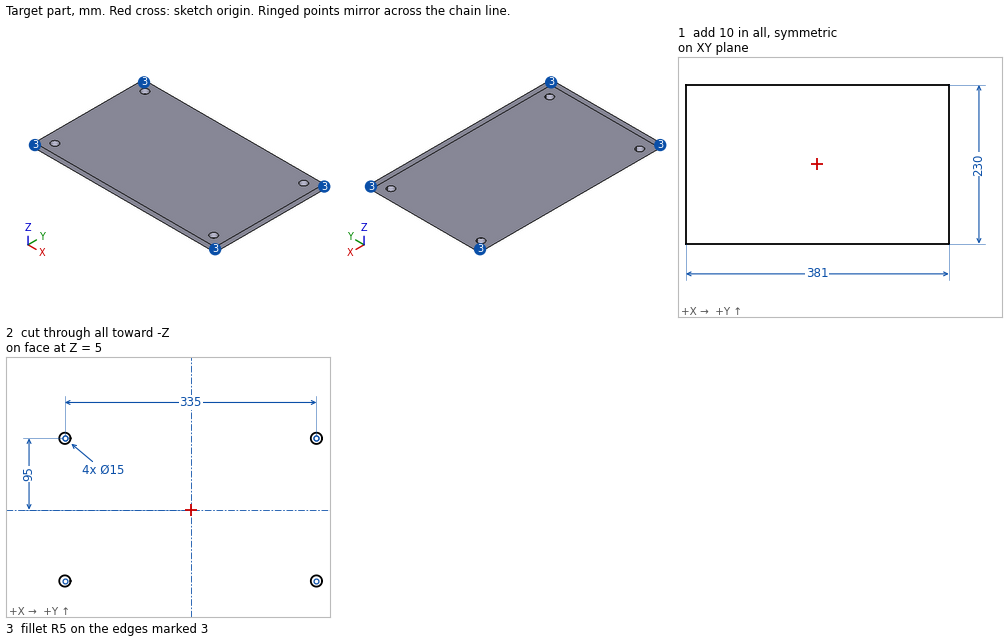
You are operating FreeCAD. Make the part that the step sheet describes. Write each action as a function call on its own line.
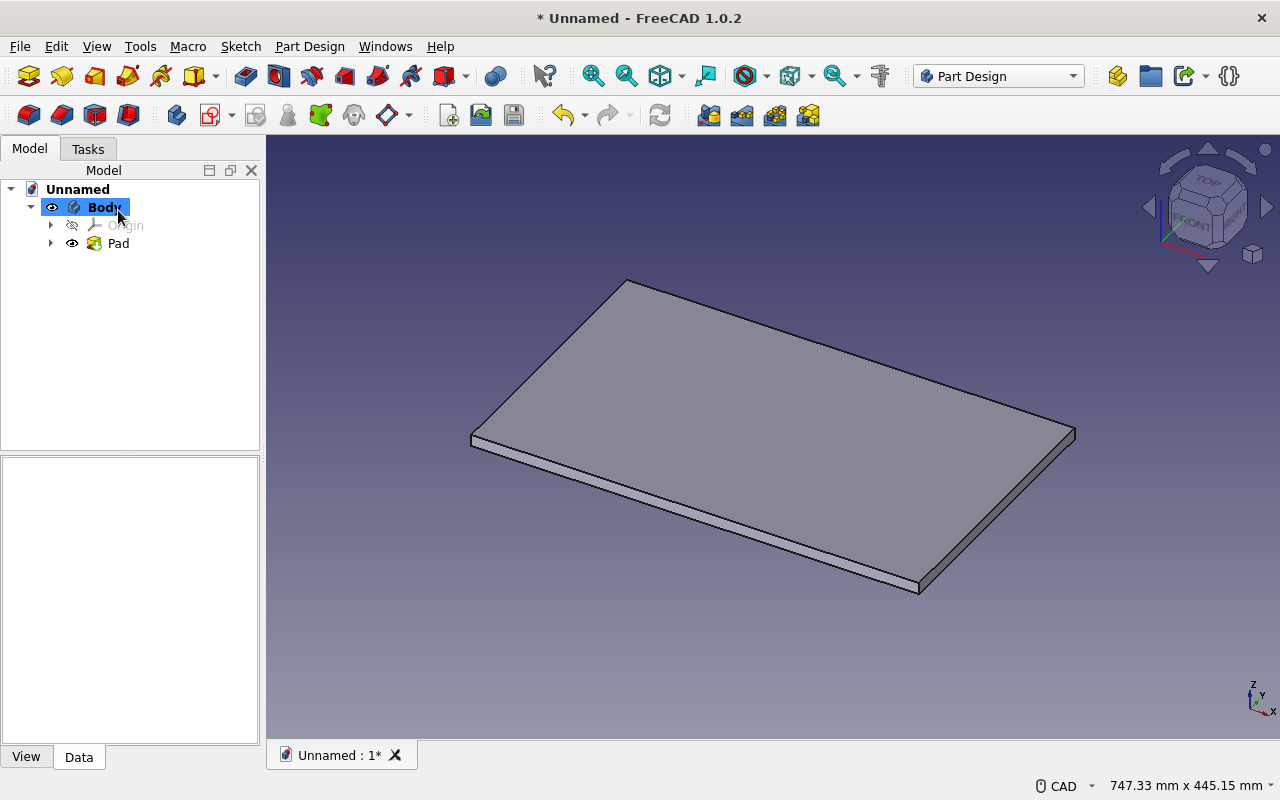
click(837, 452)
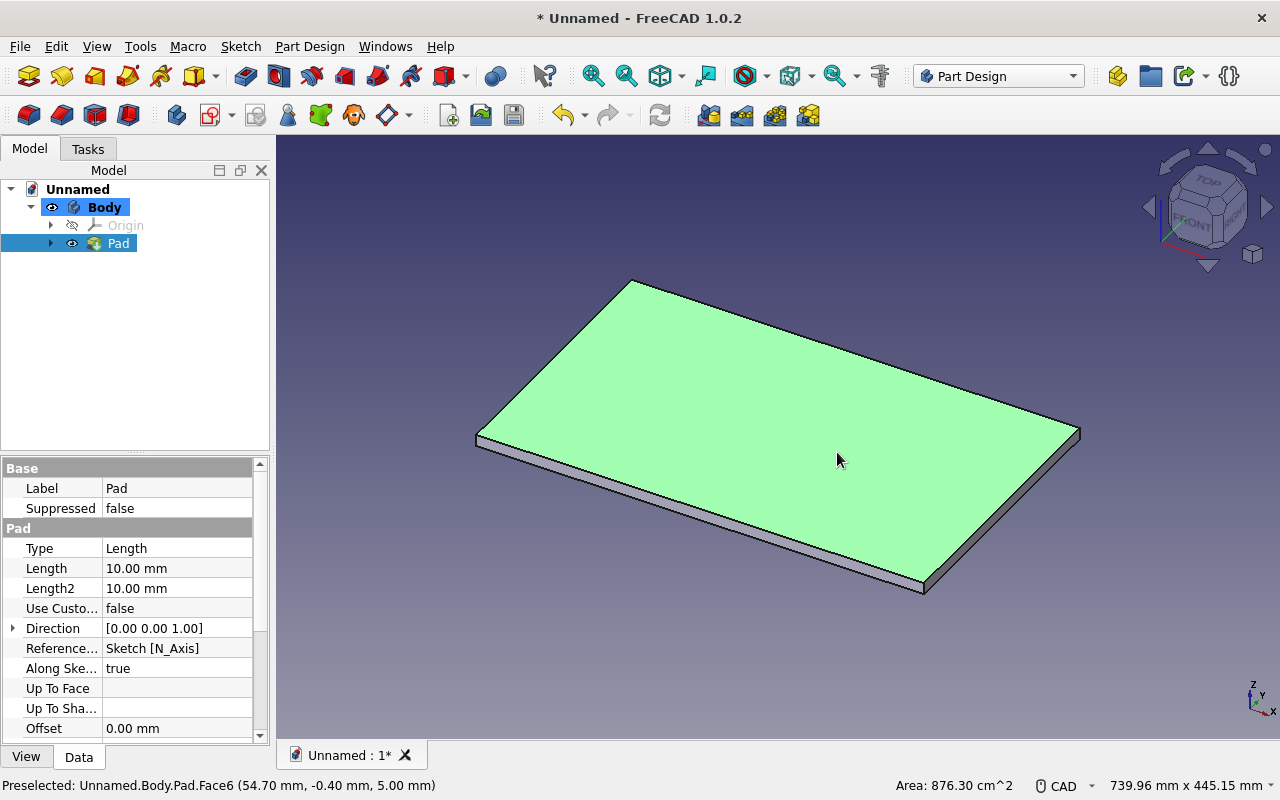
click(210, 116)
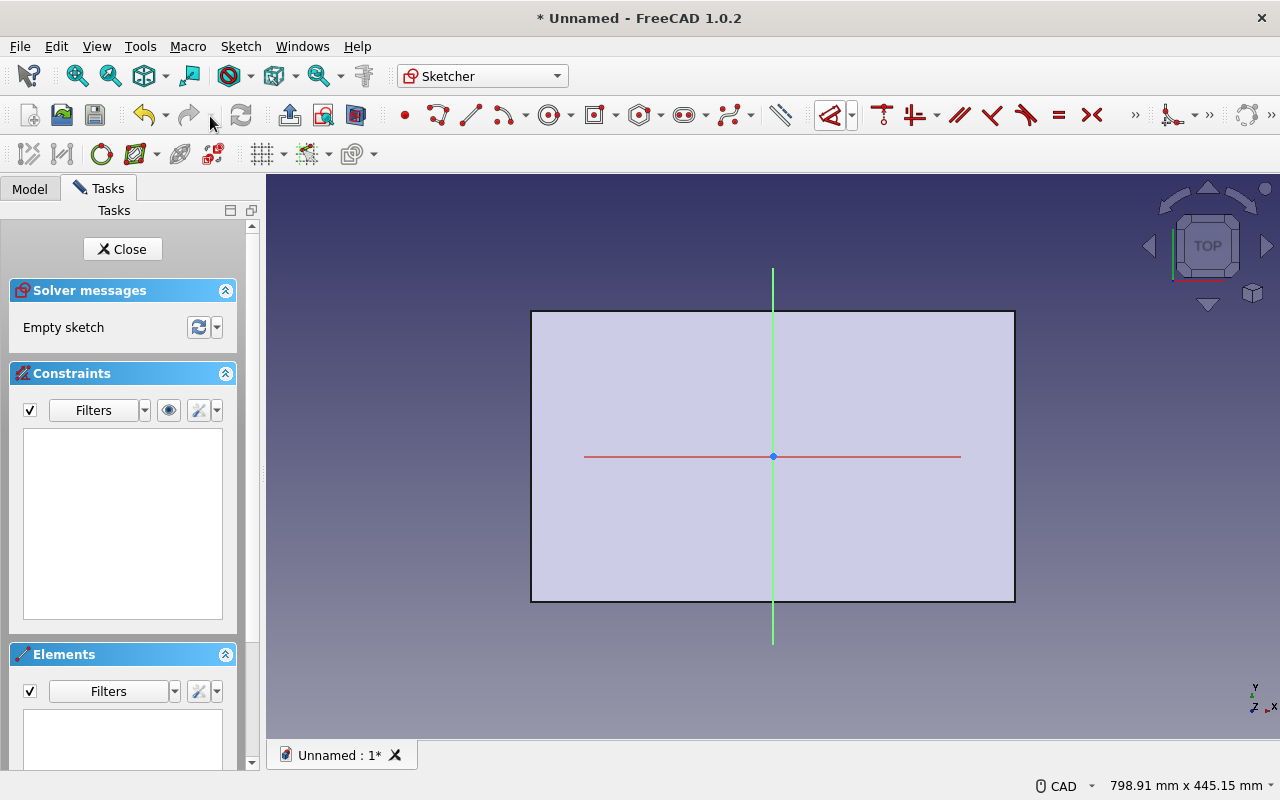
click(548, 116)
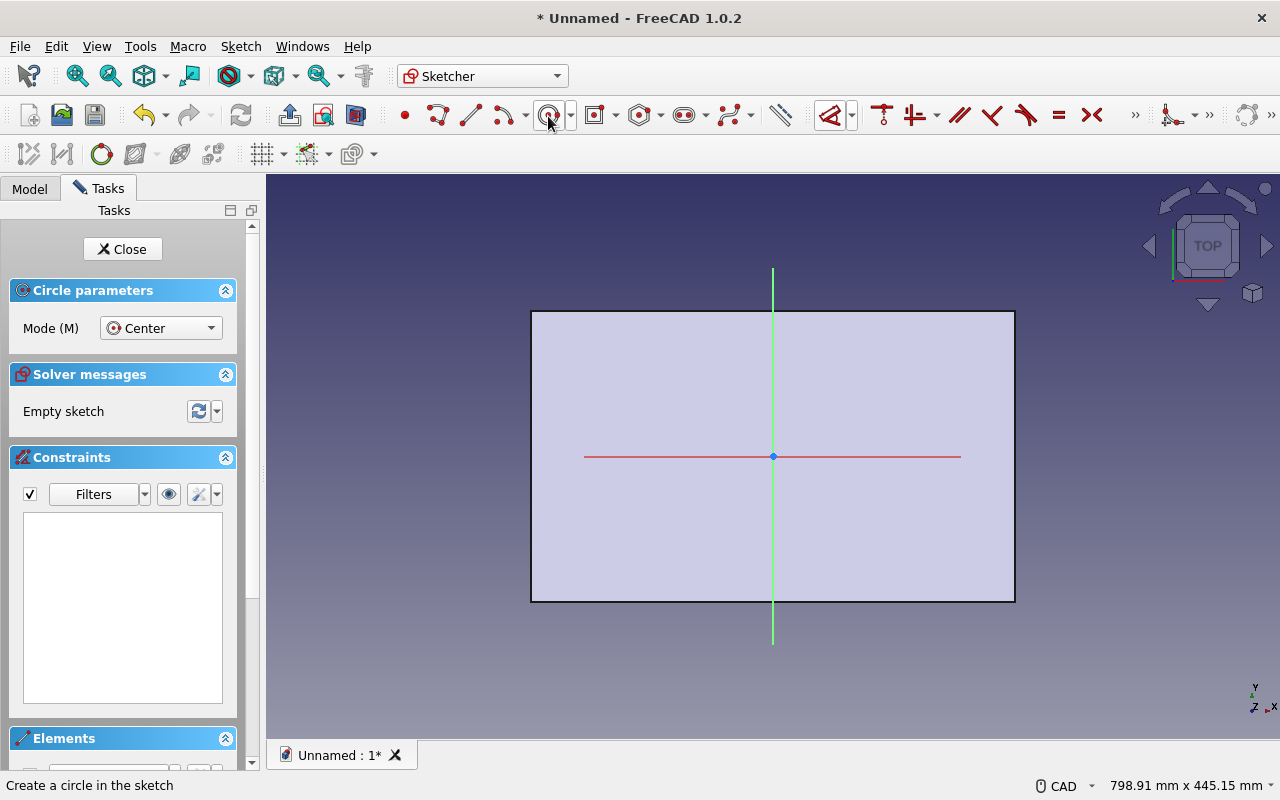
scroll(560, 336, up, 5)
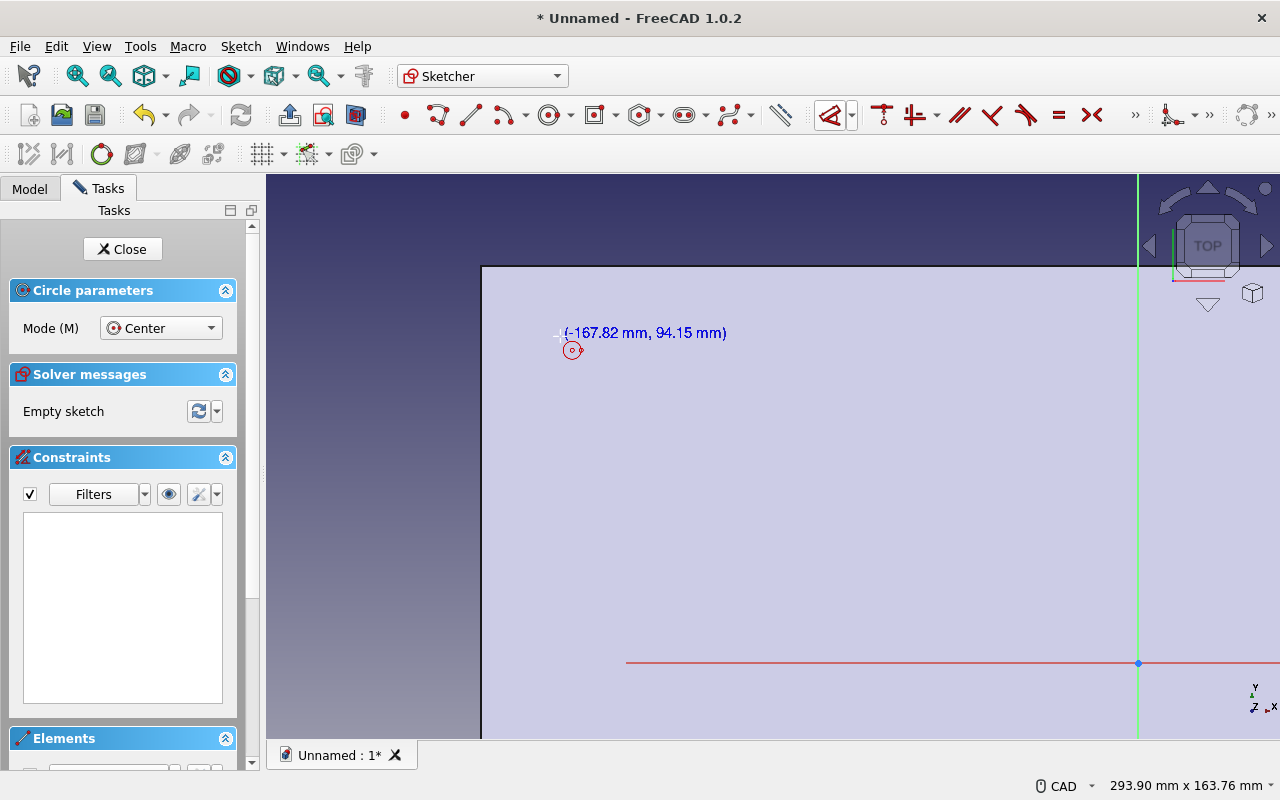
click(561, 335)
click(579, 317)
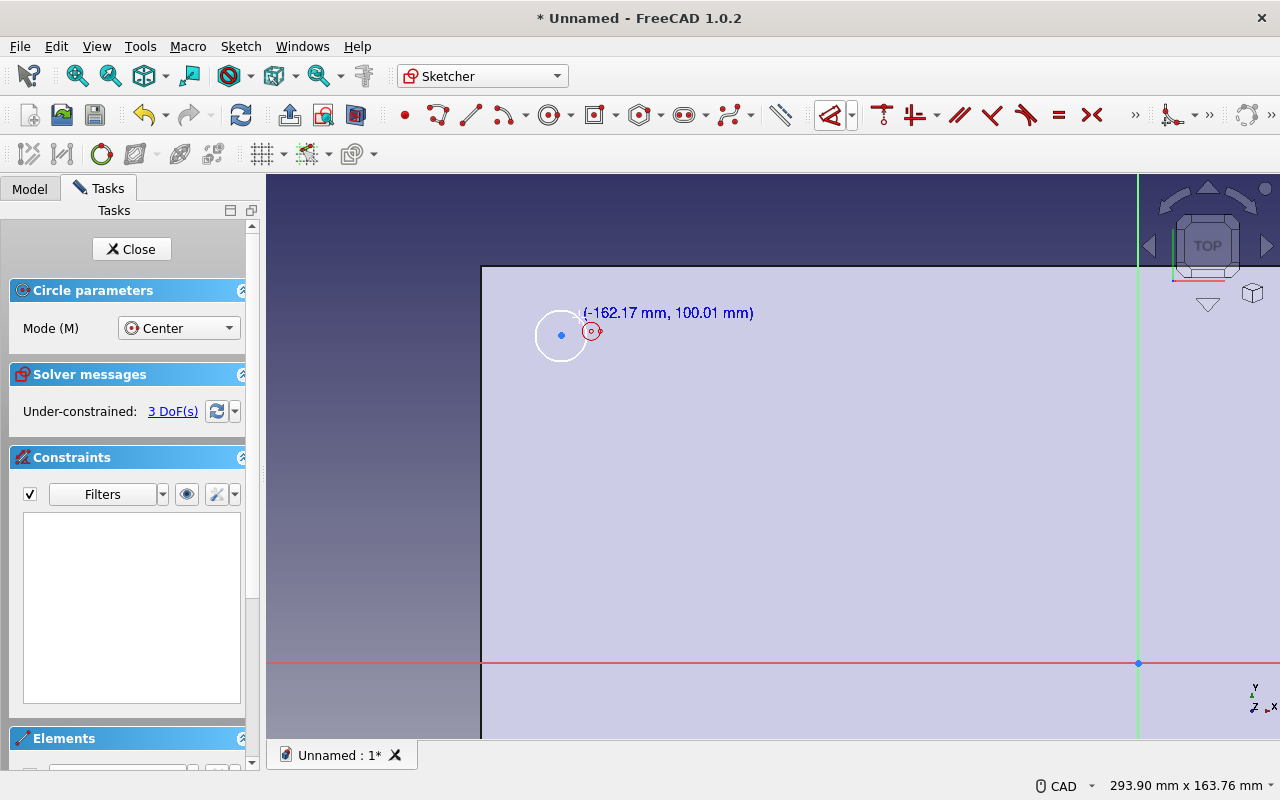
scroll(350, 288, down, 4)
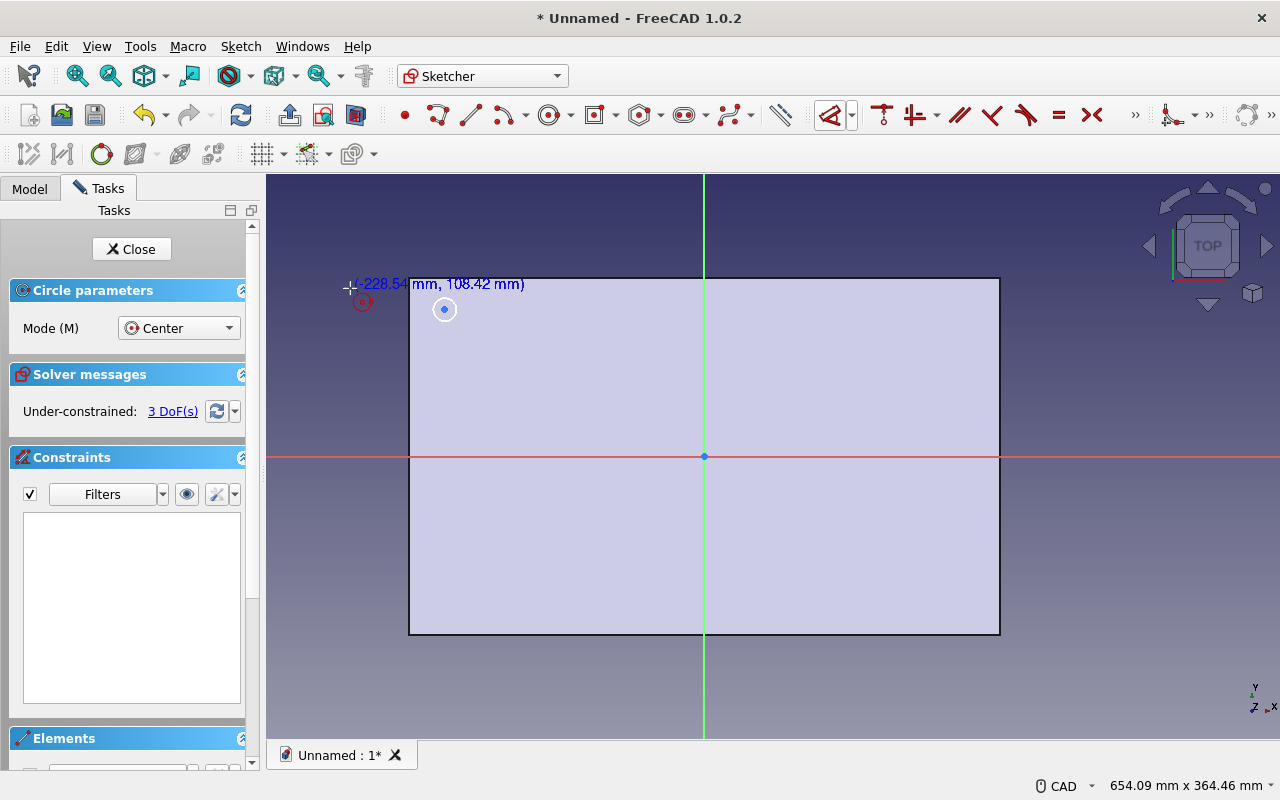
scroll(964, 309, up, 4)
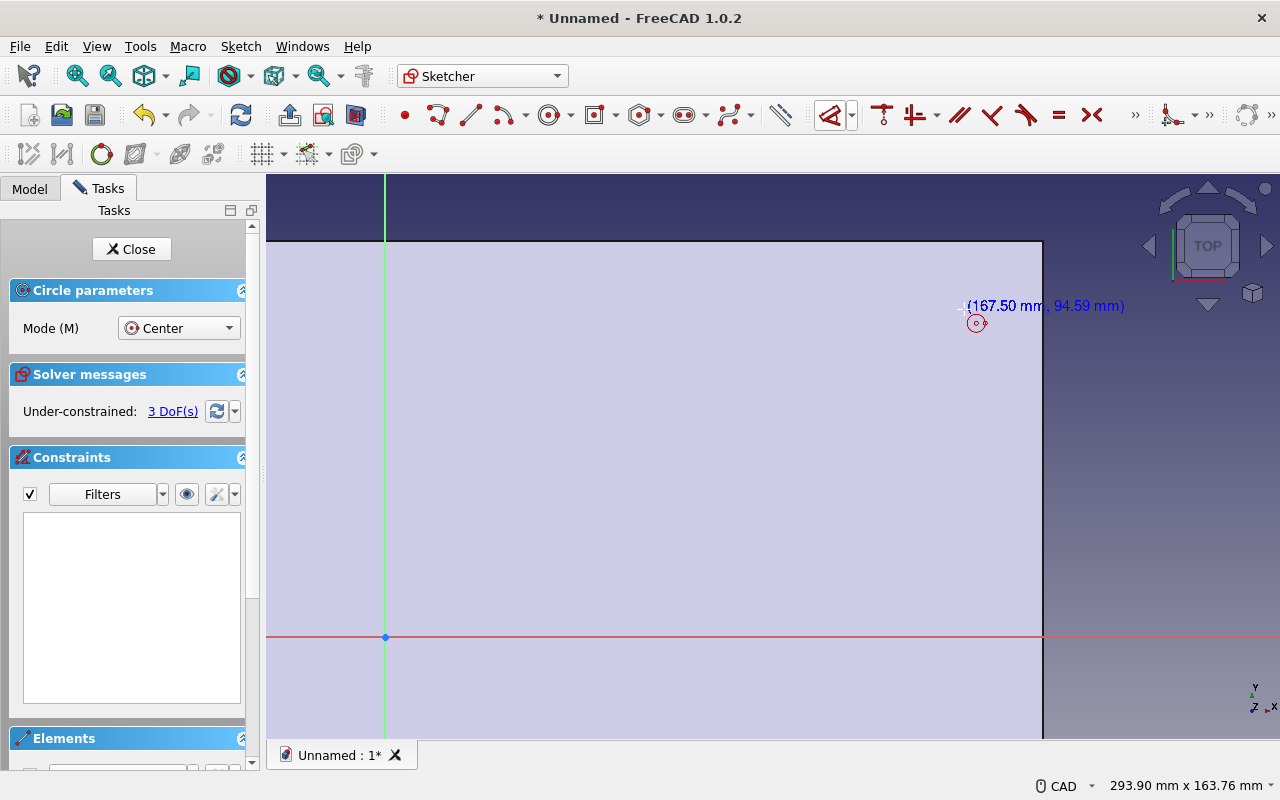
click(963, 310)
click(981, 291)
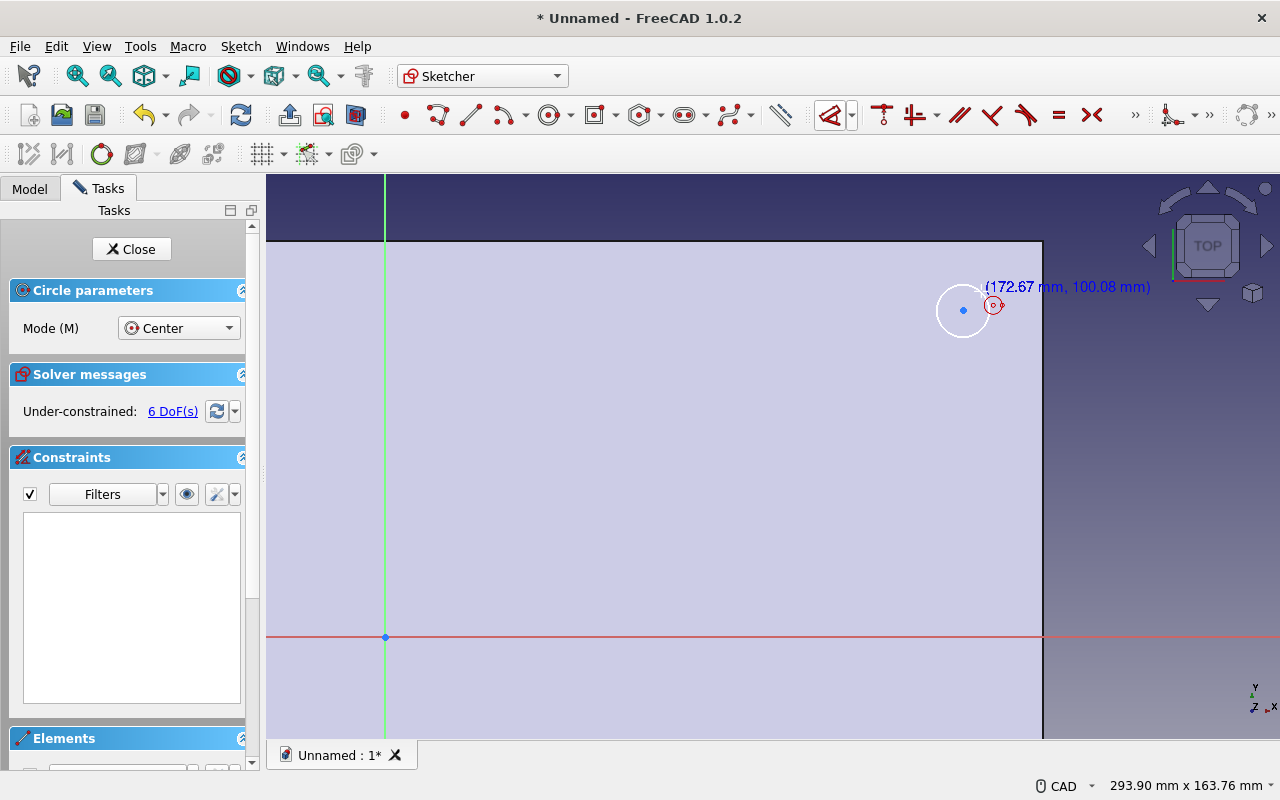
scroll(965, 309, down, 4)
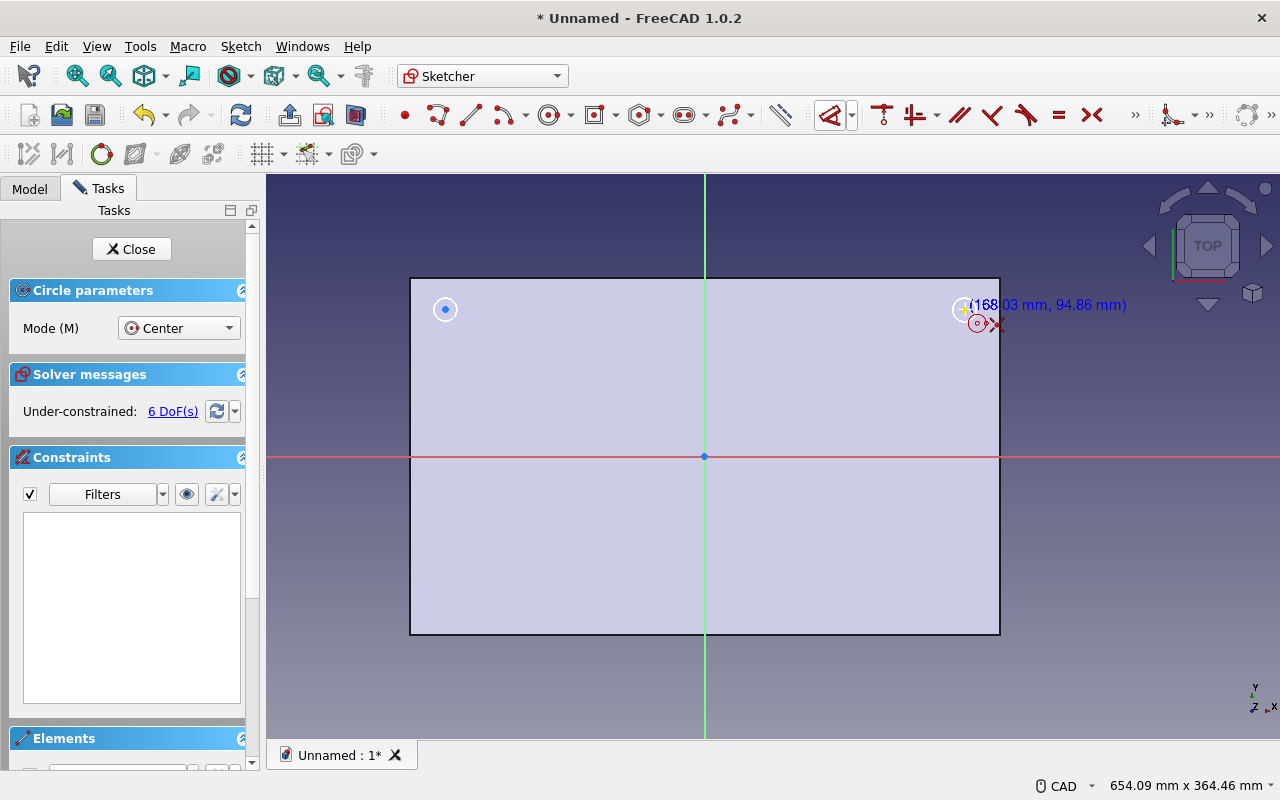
scroll(965, 604, up, 4)